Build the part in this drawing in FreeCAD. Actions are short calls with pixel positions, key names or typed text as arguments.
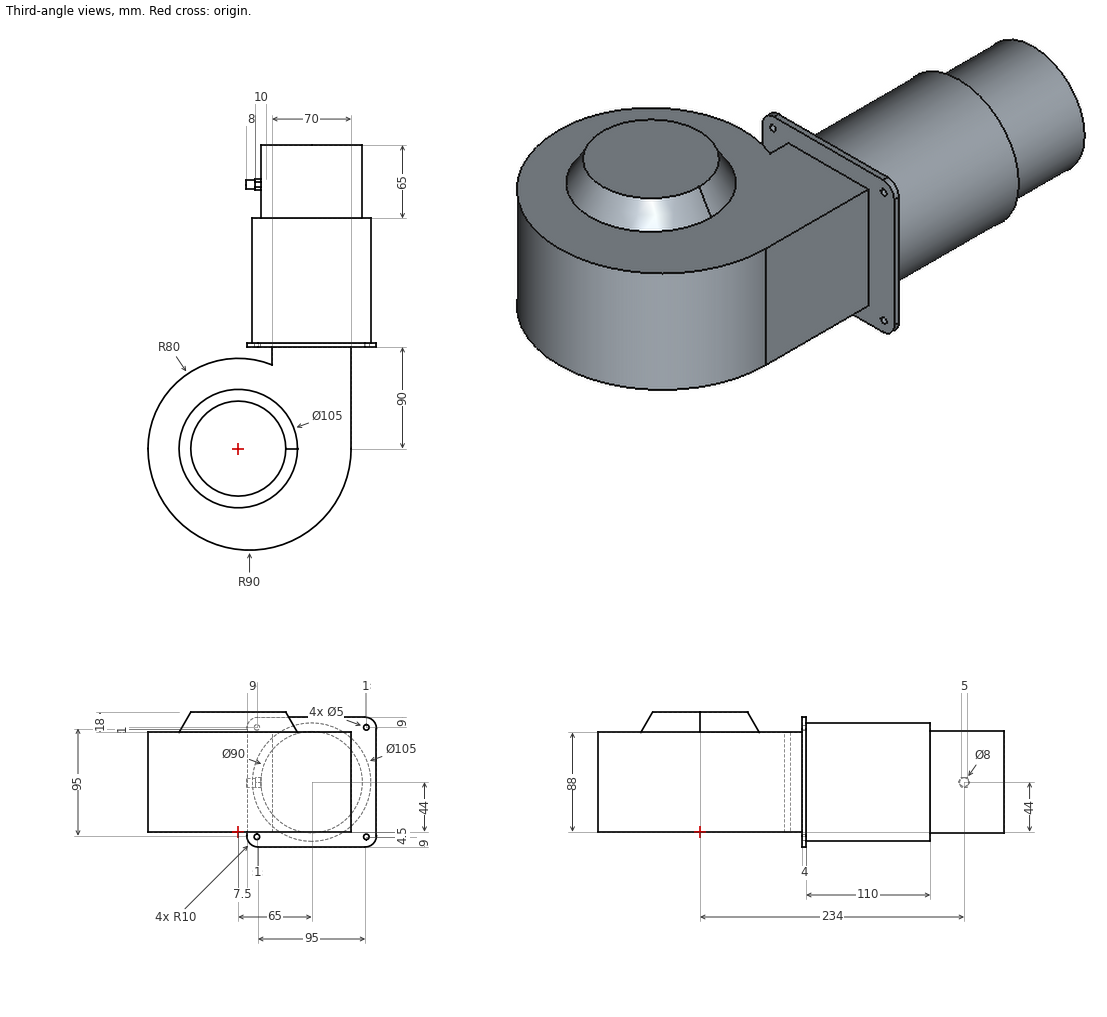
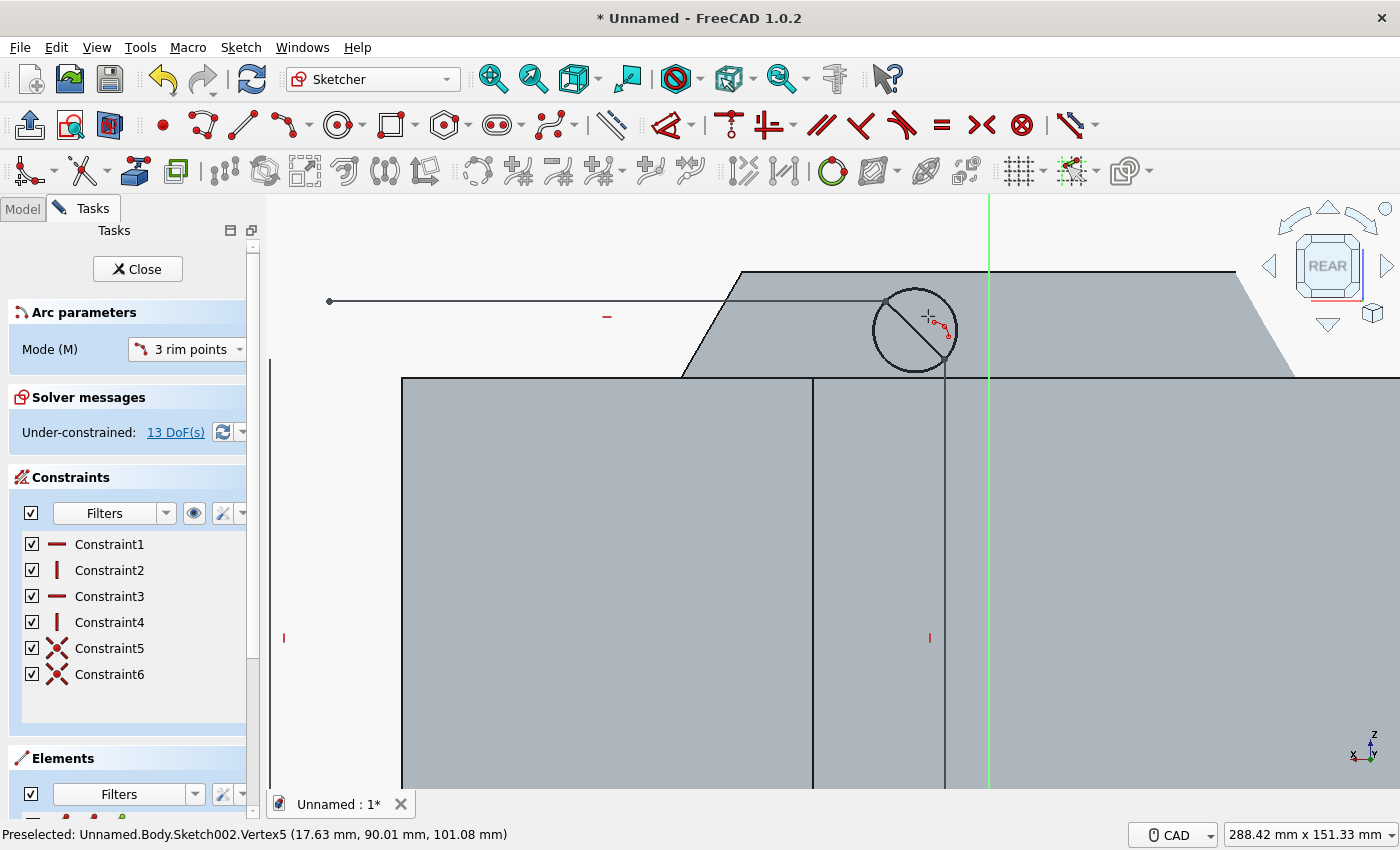
click(928, 316)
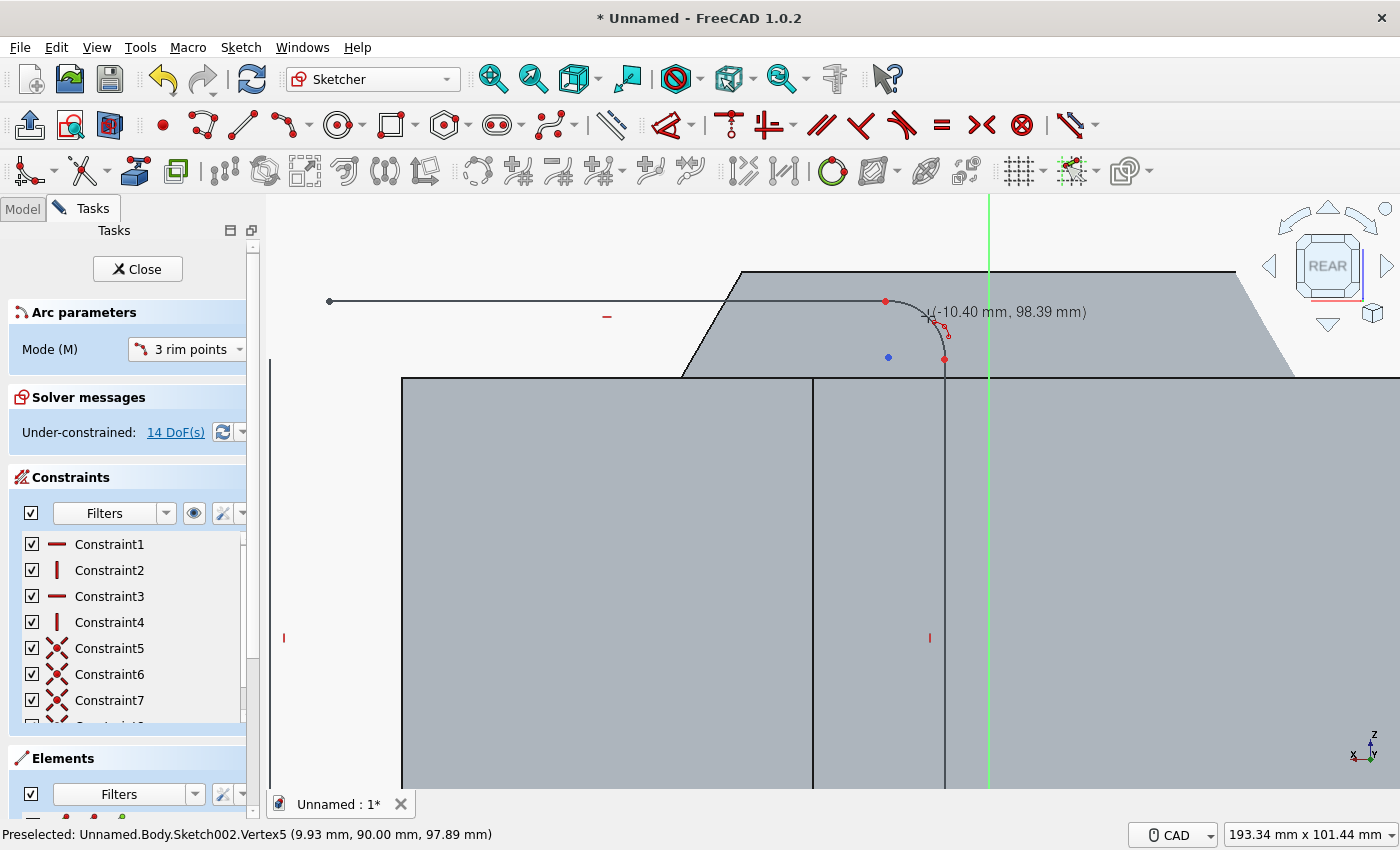
click(330, 301)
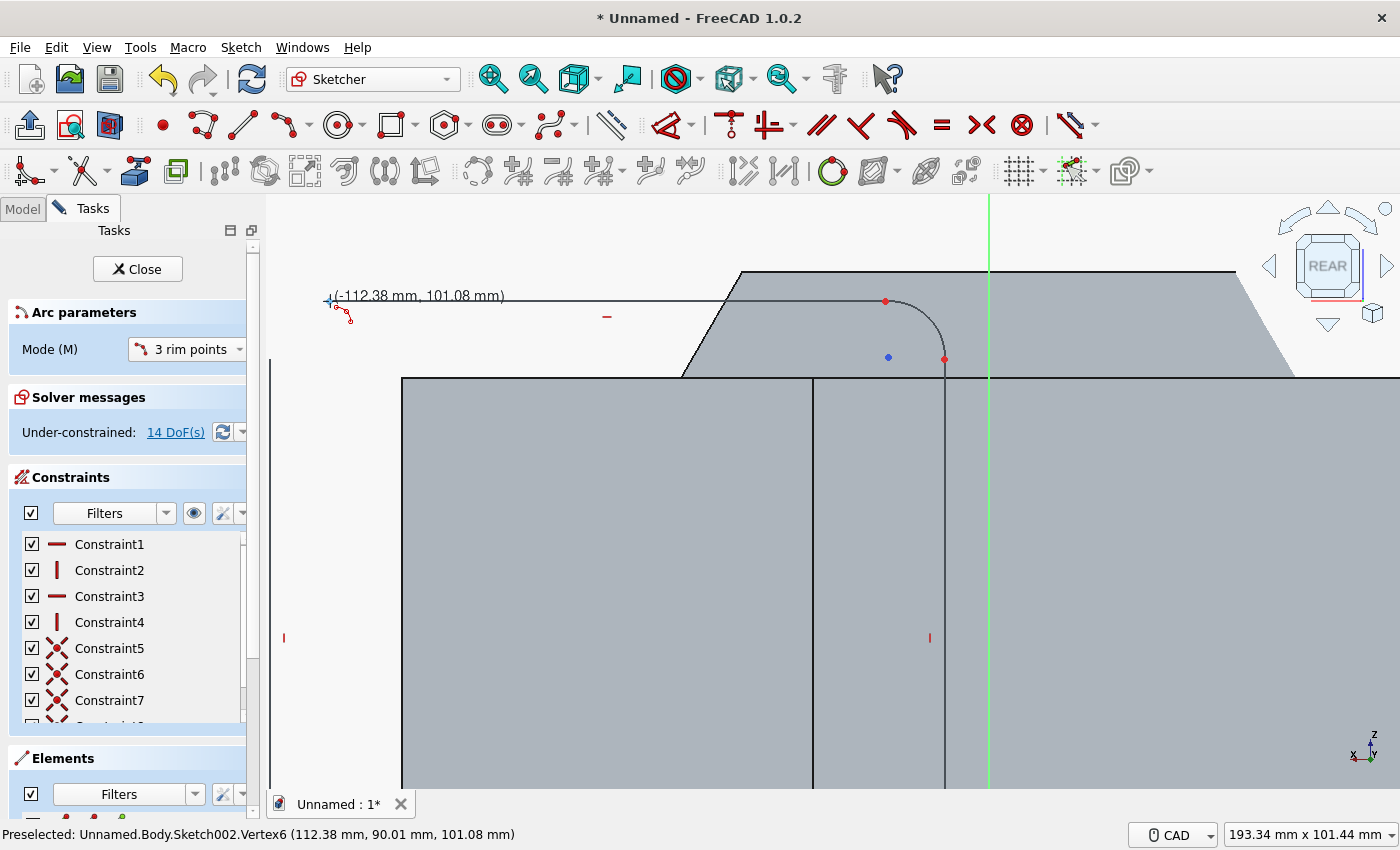
scroll(928, 316, down, 3)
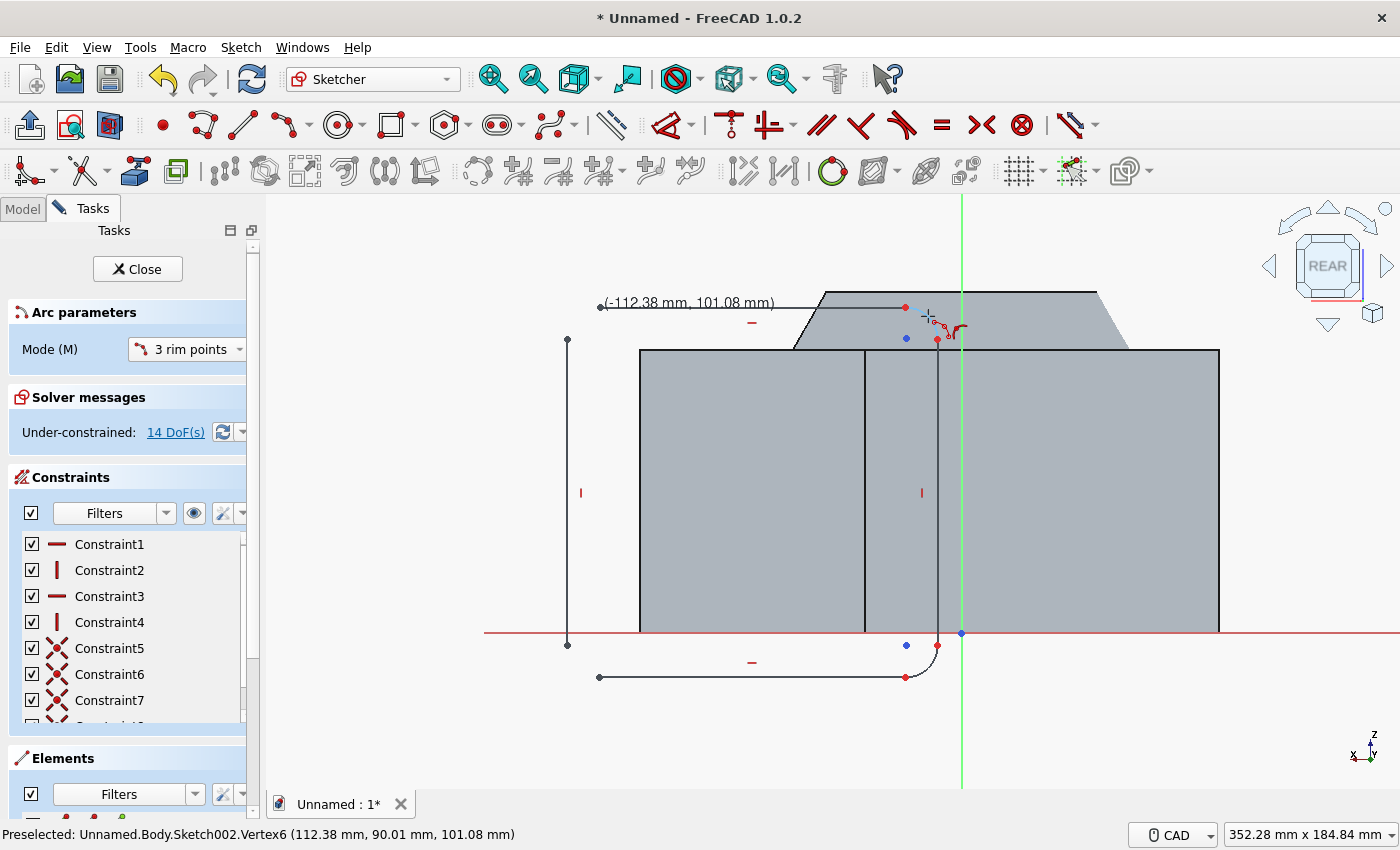
click(567, 340)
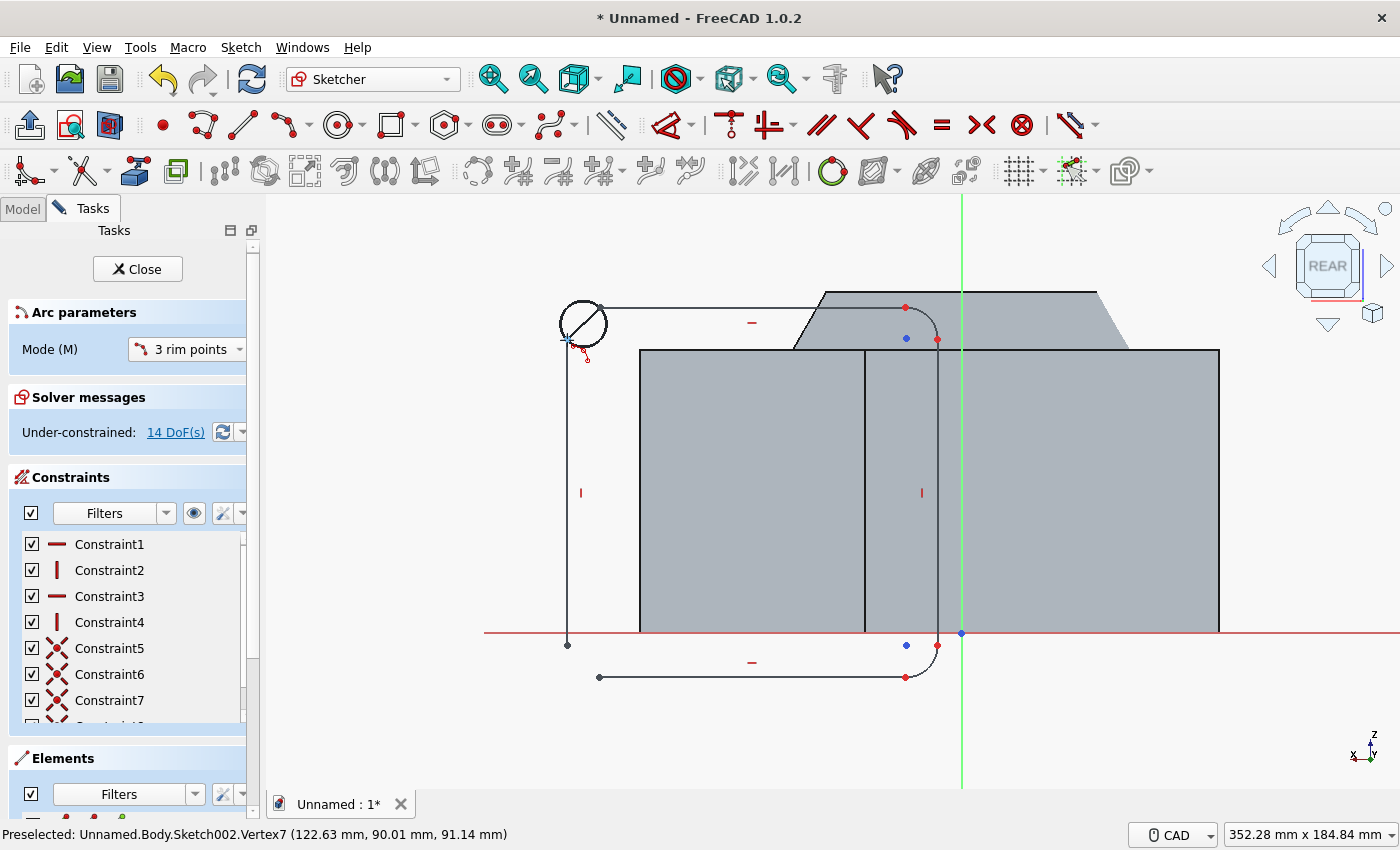
scroll(577, 316, up, 3)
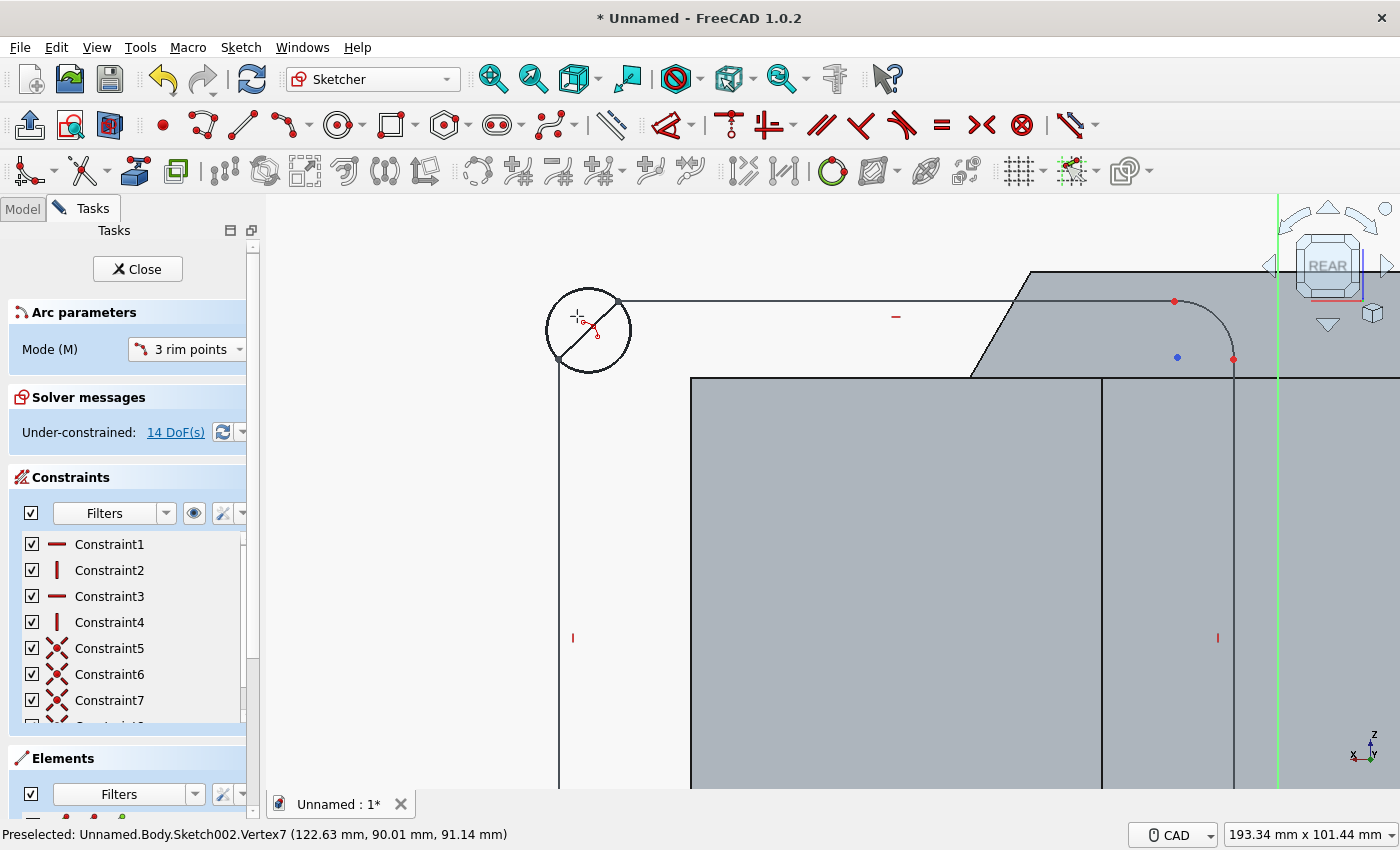
click(577, 316)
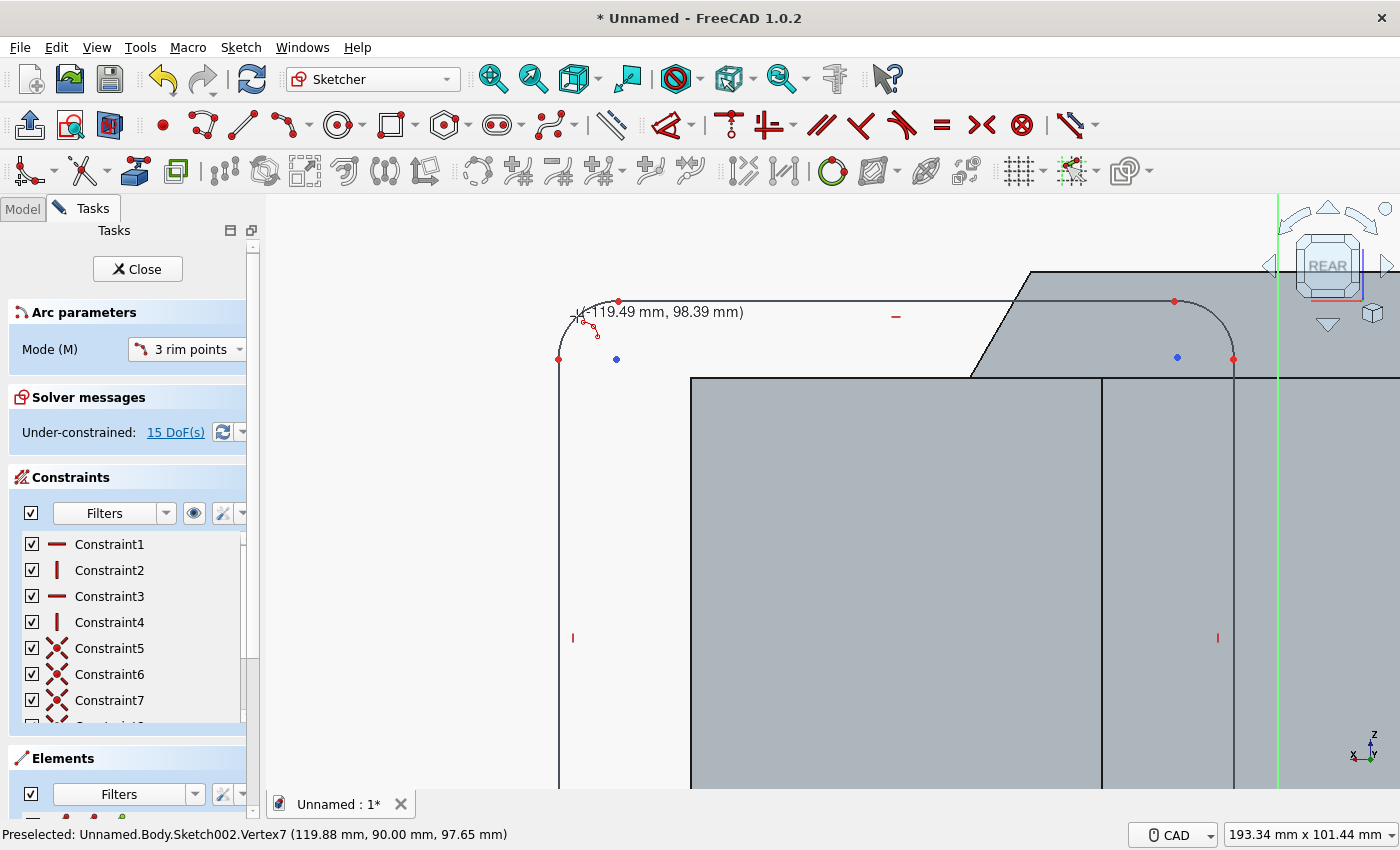
scroll(577, 316, down, 3)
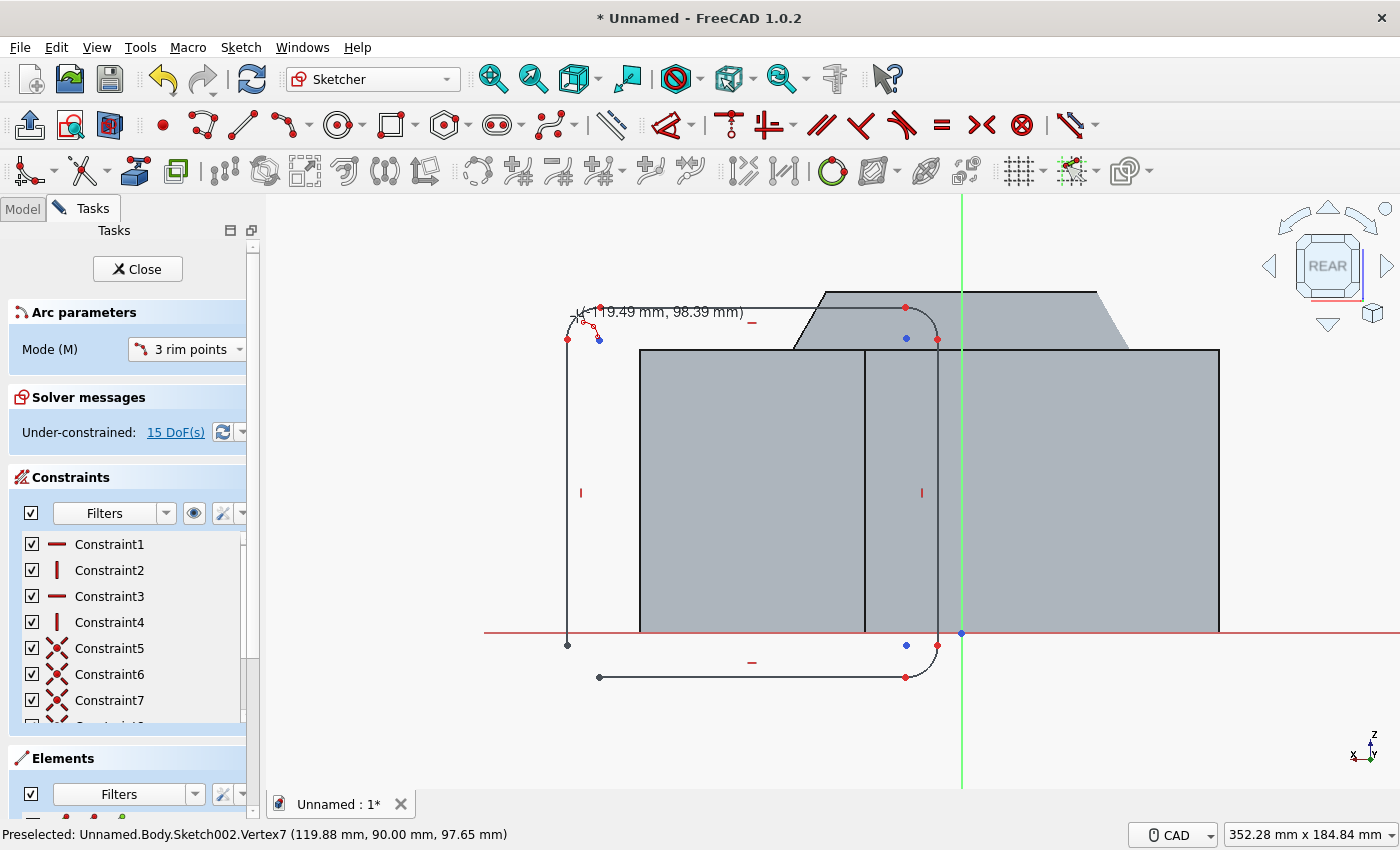
scroll(567, 645, up, 2)